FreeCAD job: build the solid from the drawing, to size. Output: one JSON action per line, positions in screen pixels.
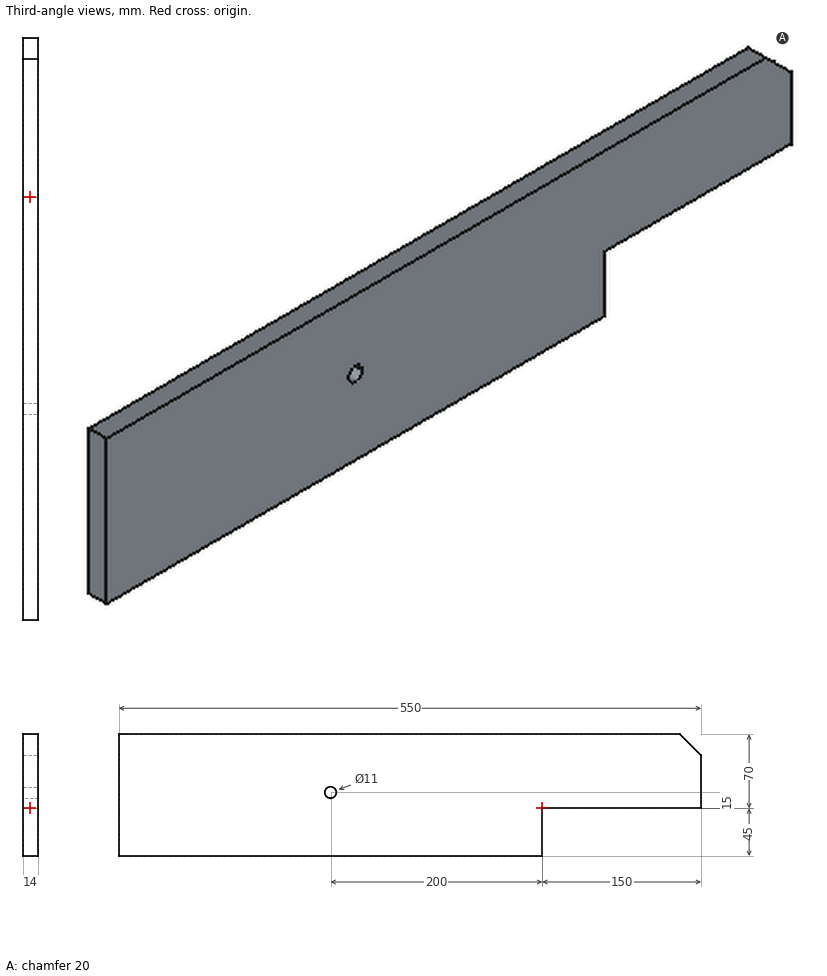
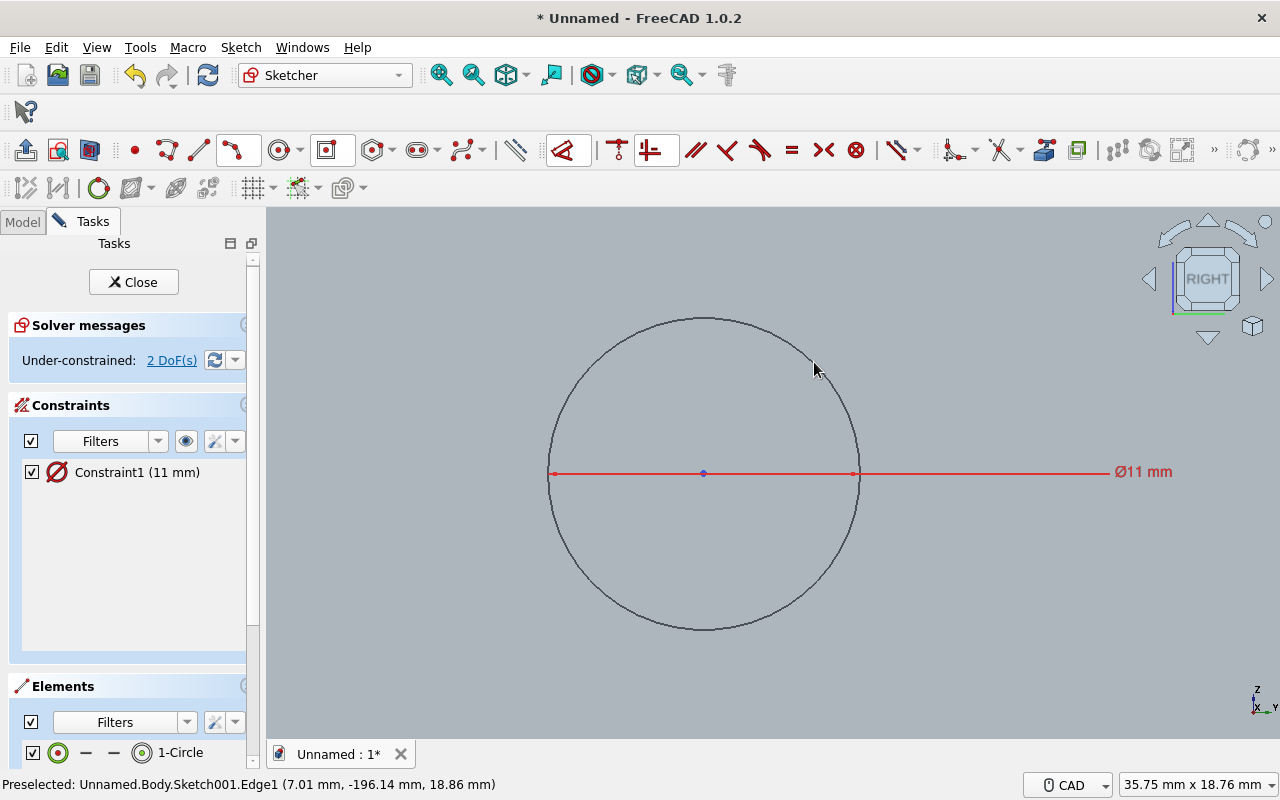
{"action": "left_click", "coordinate": [704, 474]}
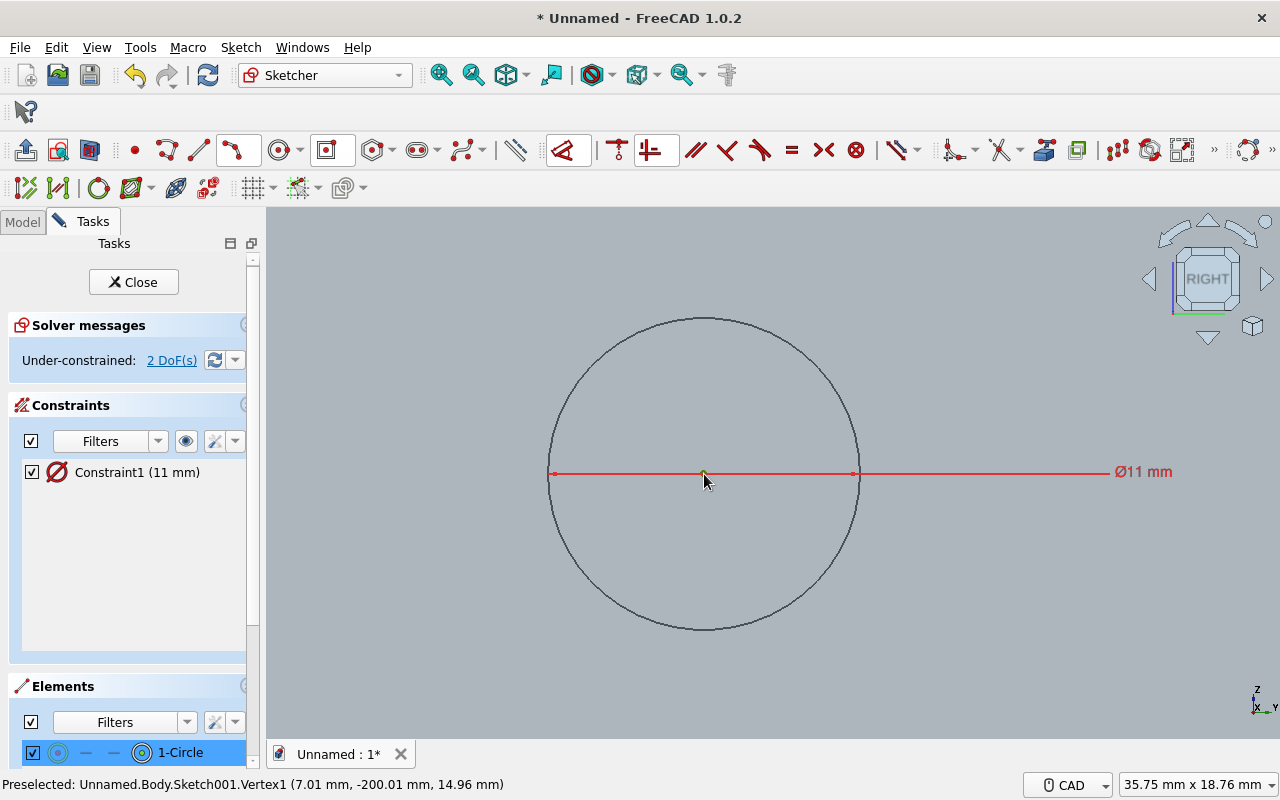
{"action": "key", "text": "i"}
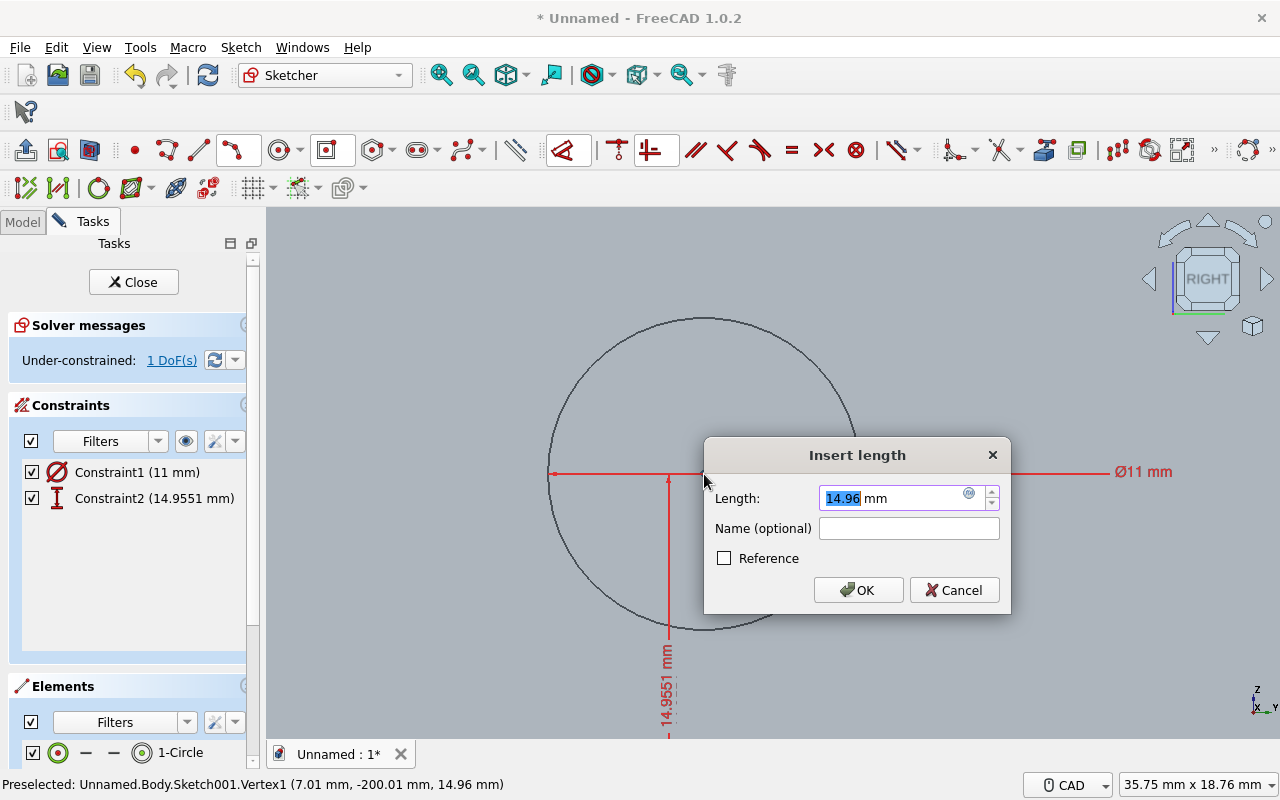
{"action": "type", "text": "15"}
{"action": "key", "text": "Return"}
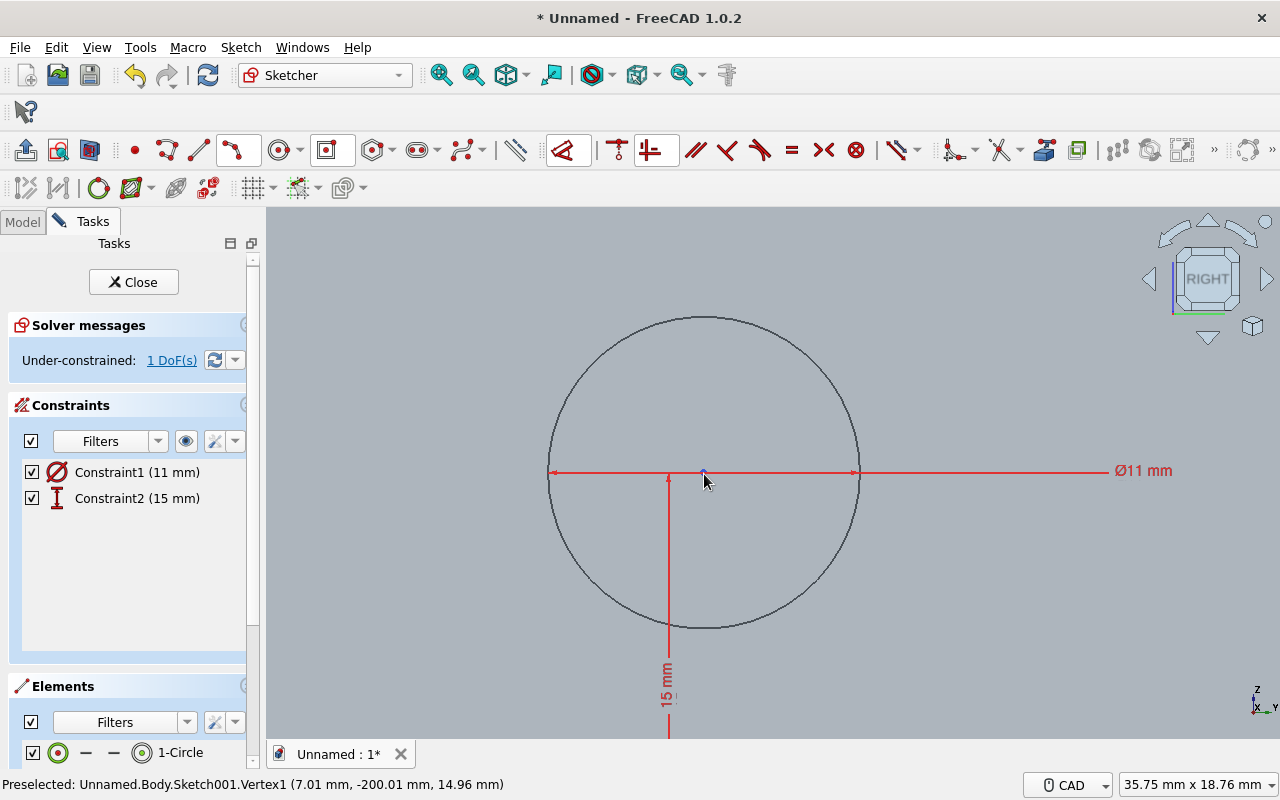
{"action": "left_click", "coordinate": [704, 473]}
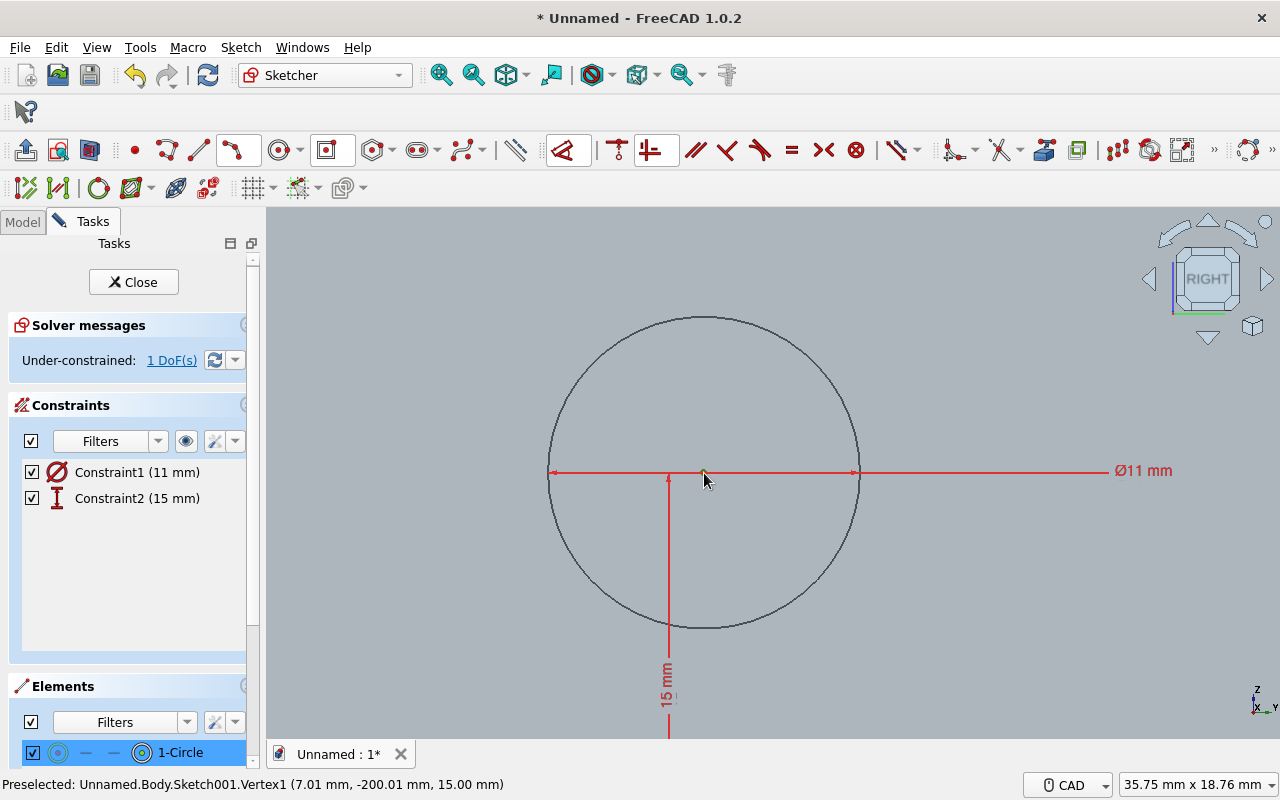
{"action": "key", "text": "l"}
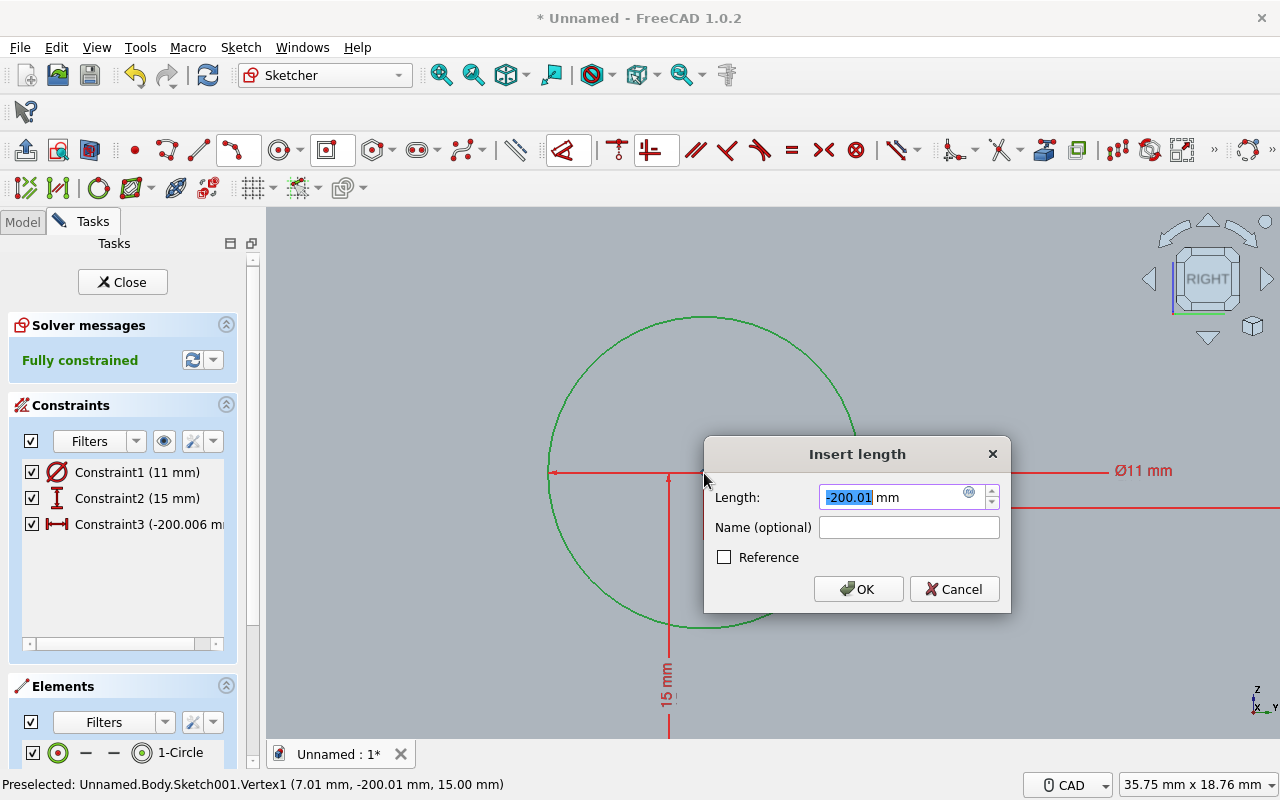
{"action": "type", "text": "-200"}
{"action": "key", "text": "Return"}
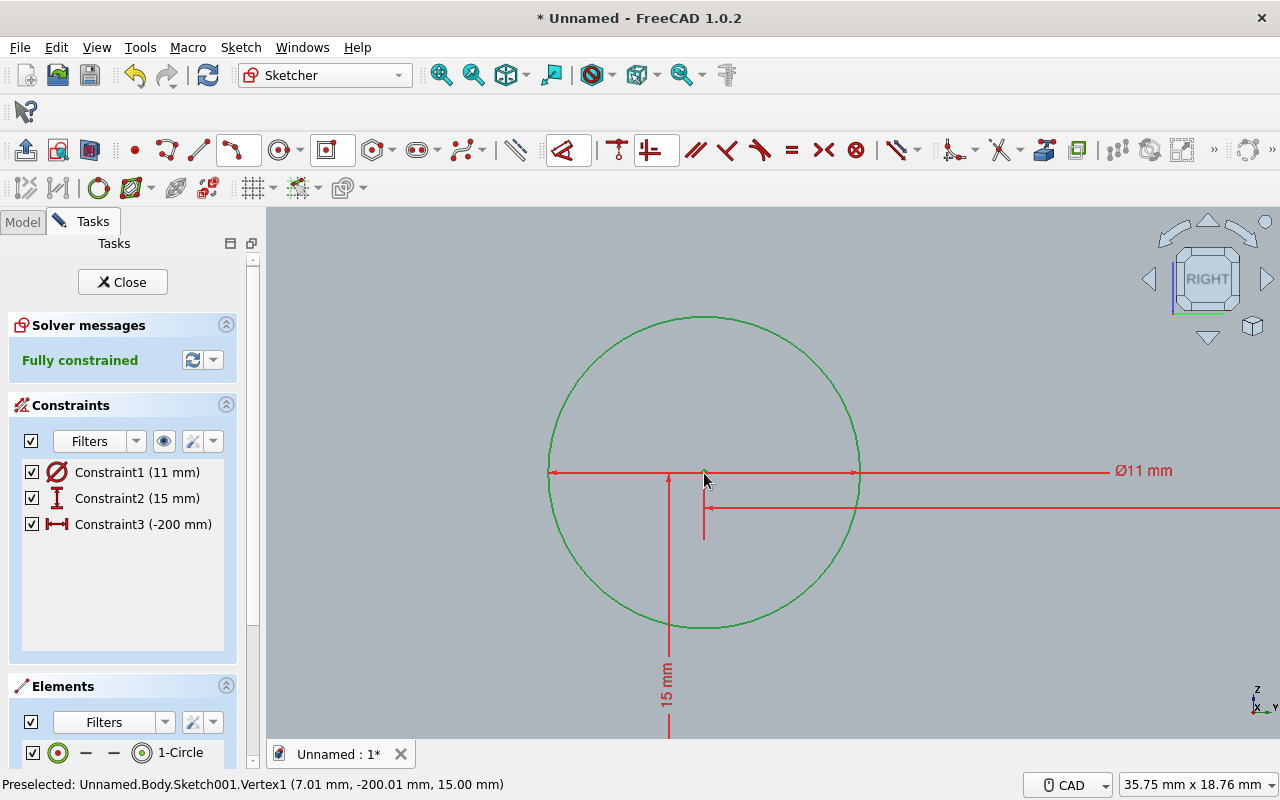
{"action": "left_click", "coordinate": [123, 282]}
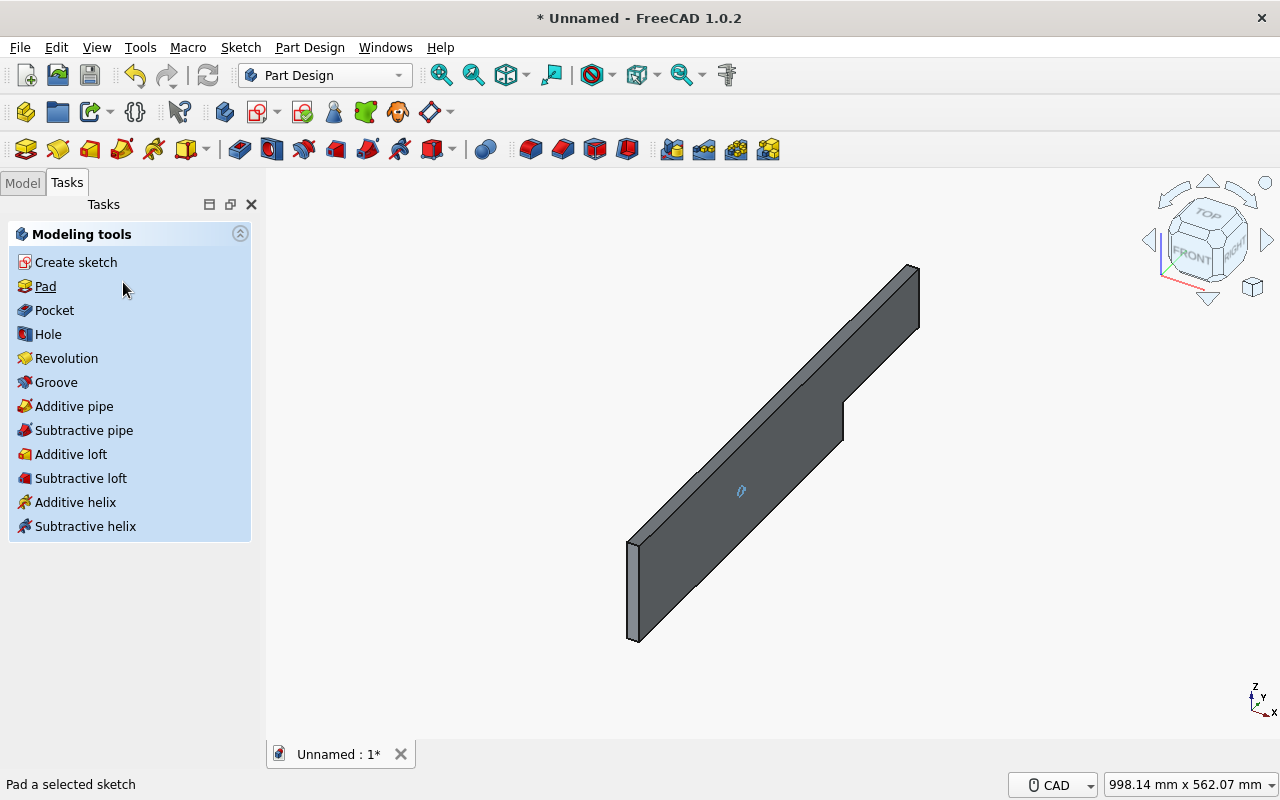
{"action": "left_click", "coordinate": [240, 150]}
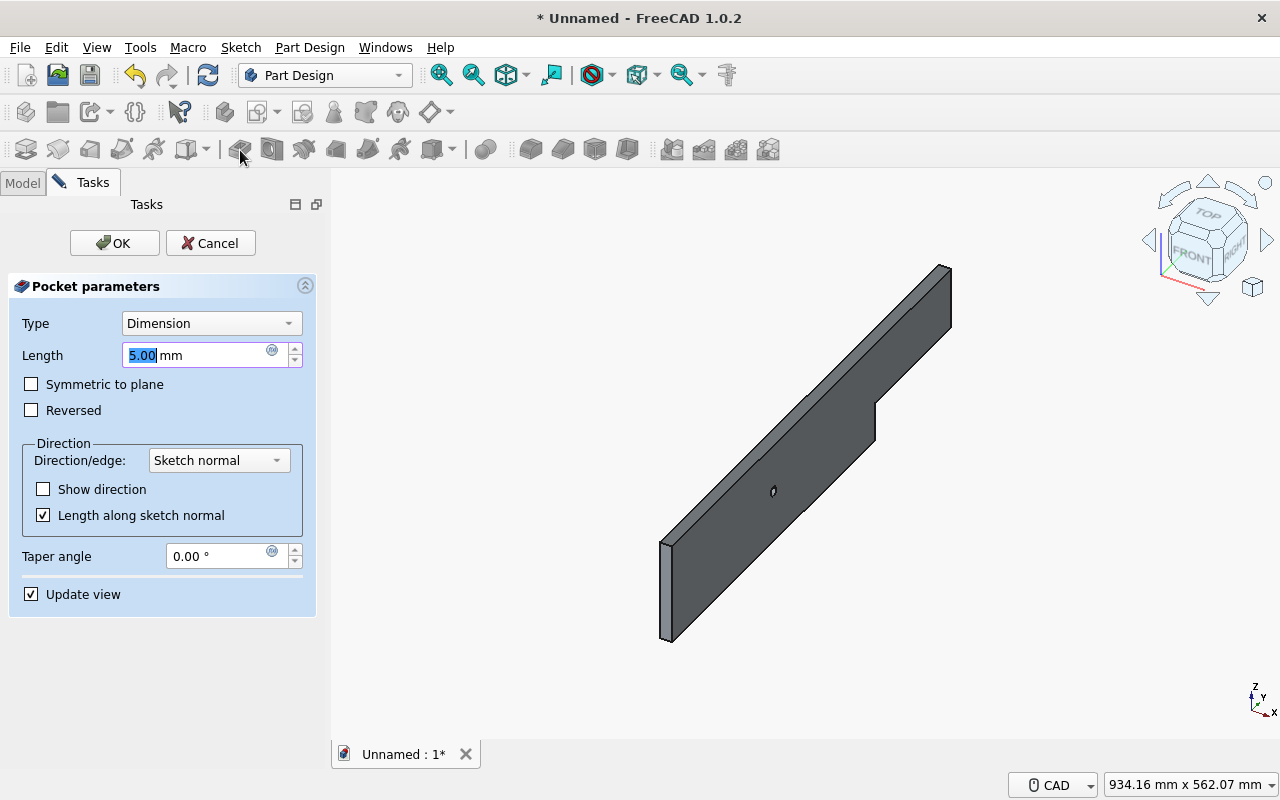
{"action": "left_click", "coordinate": [212, 324]}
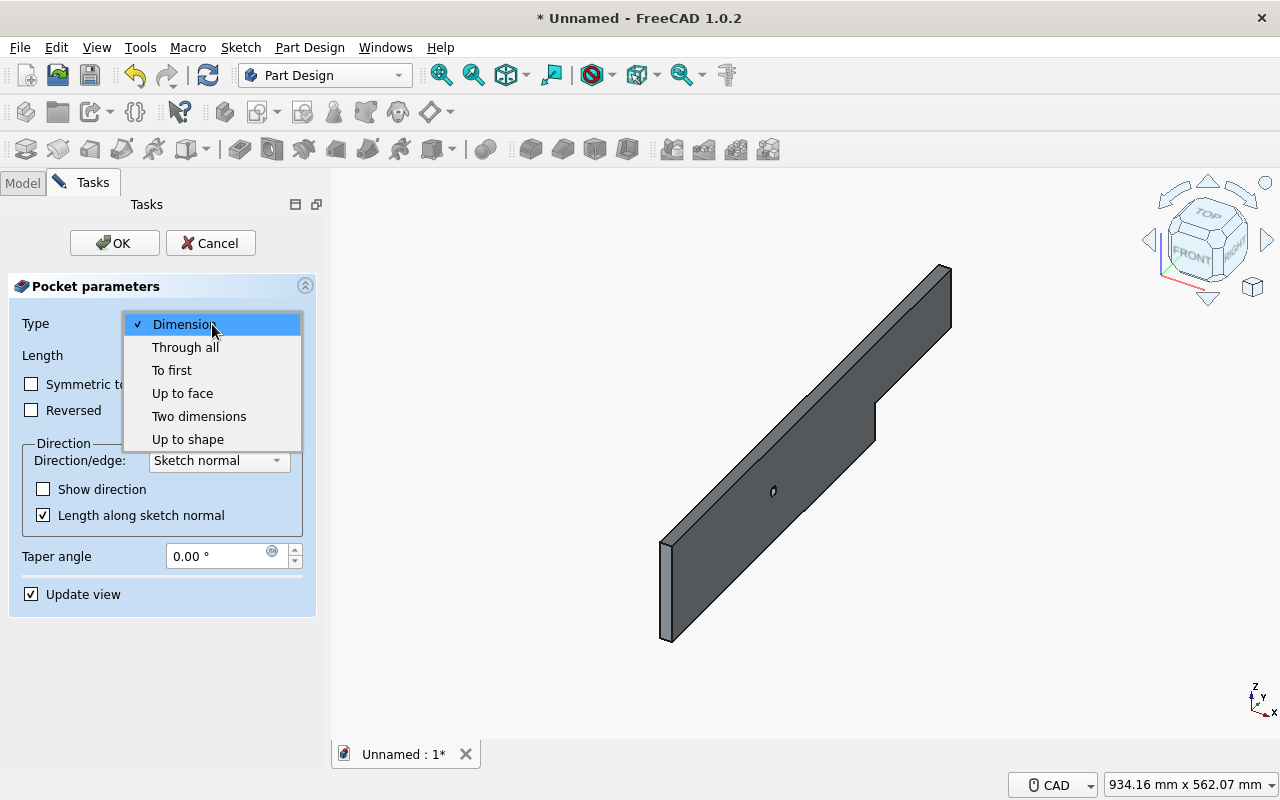
{"action": "left_click", "coordinate": [212, 370]}